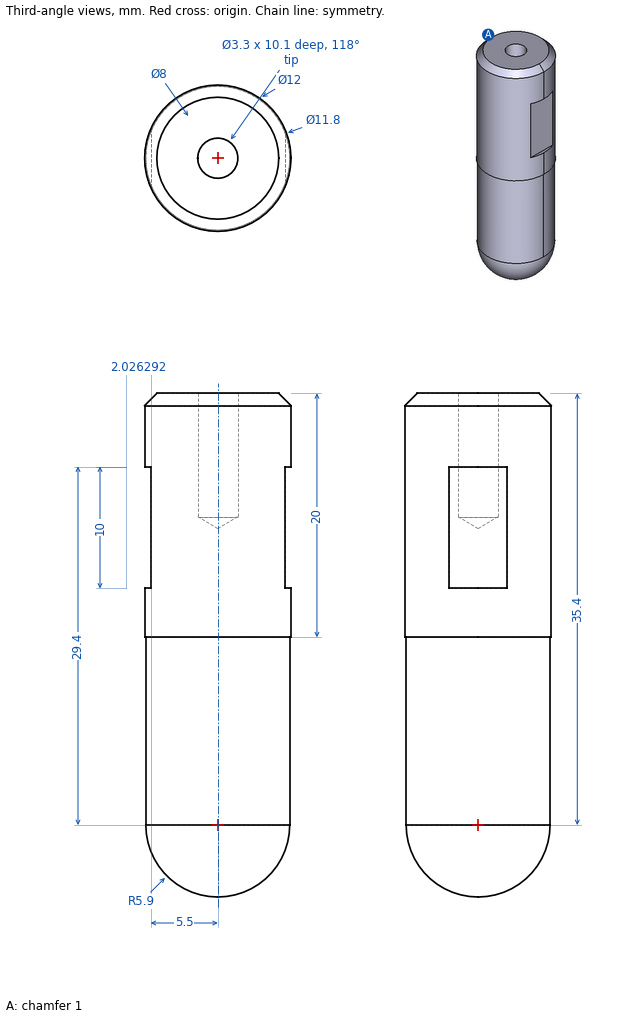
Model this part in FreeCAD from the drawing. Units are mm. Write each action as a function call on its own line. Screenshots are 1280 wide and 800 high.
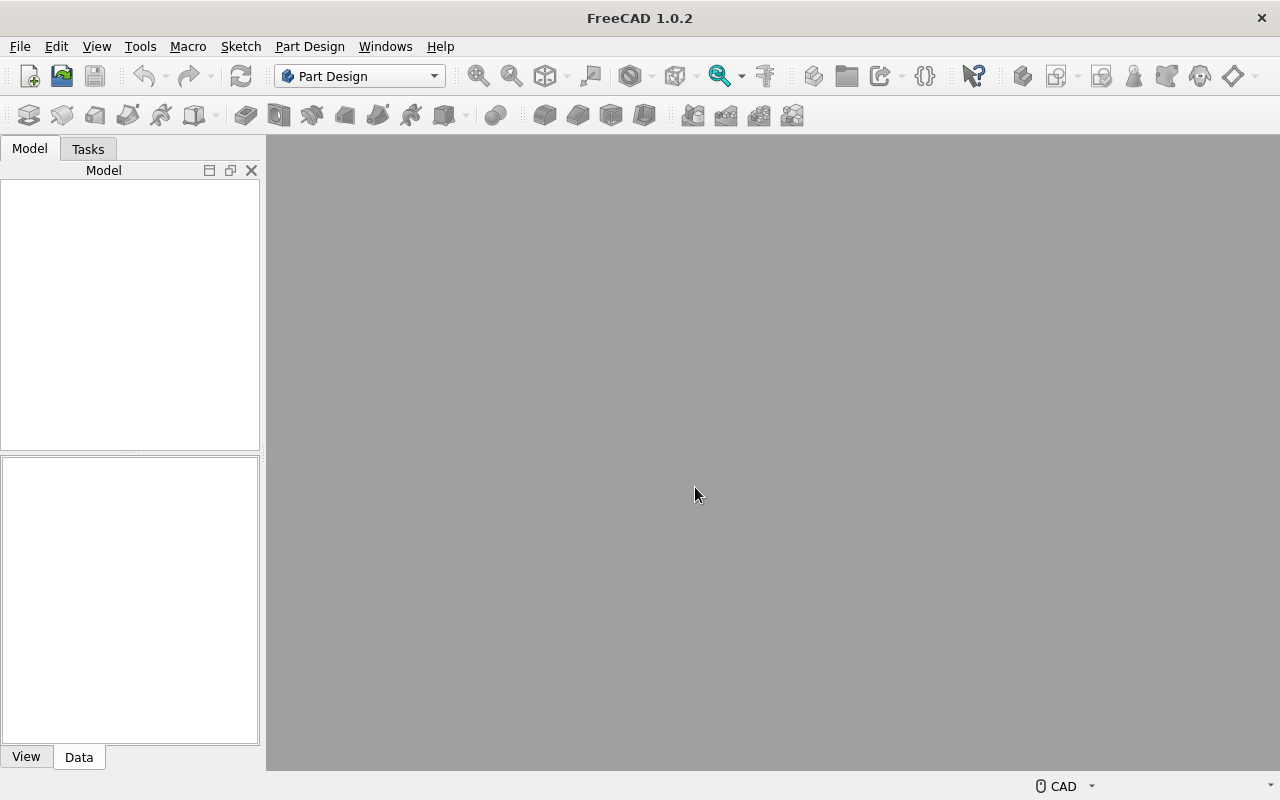
click(29, 76)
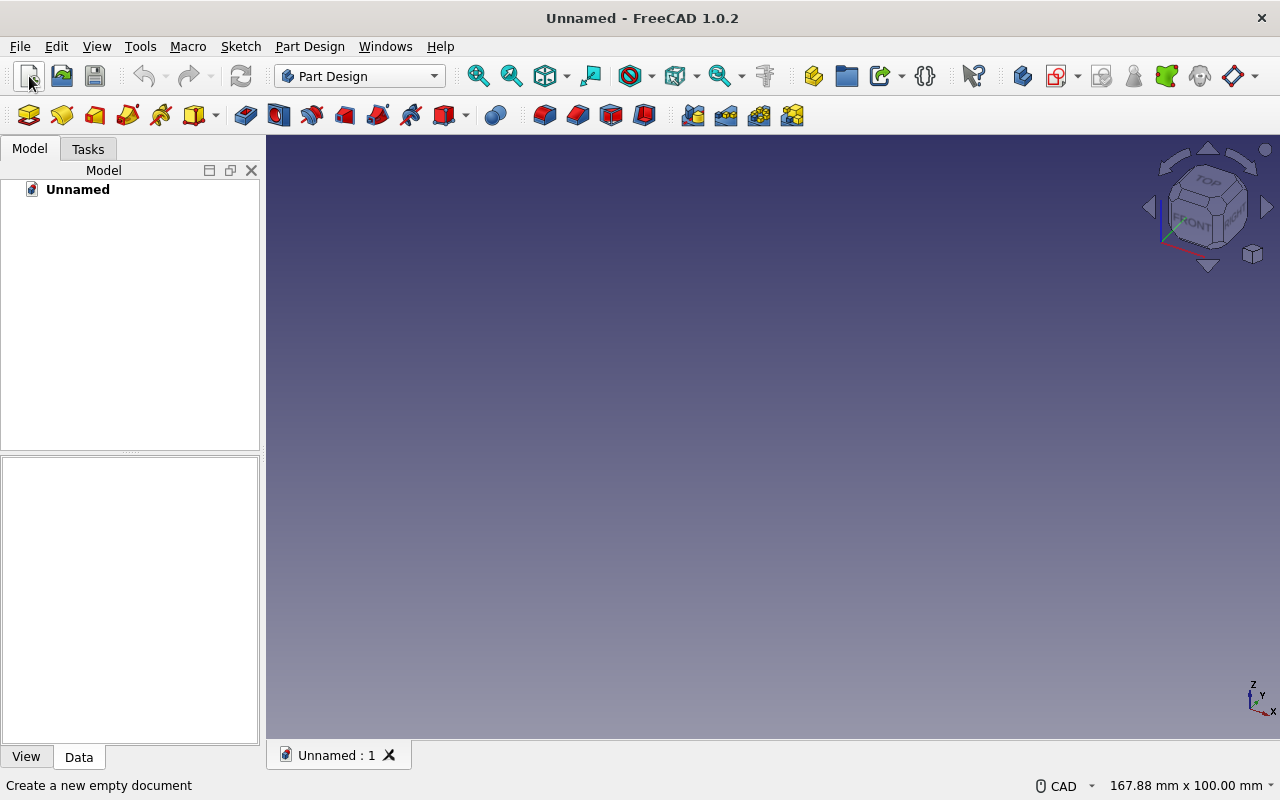
click(1056, 76)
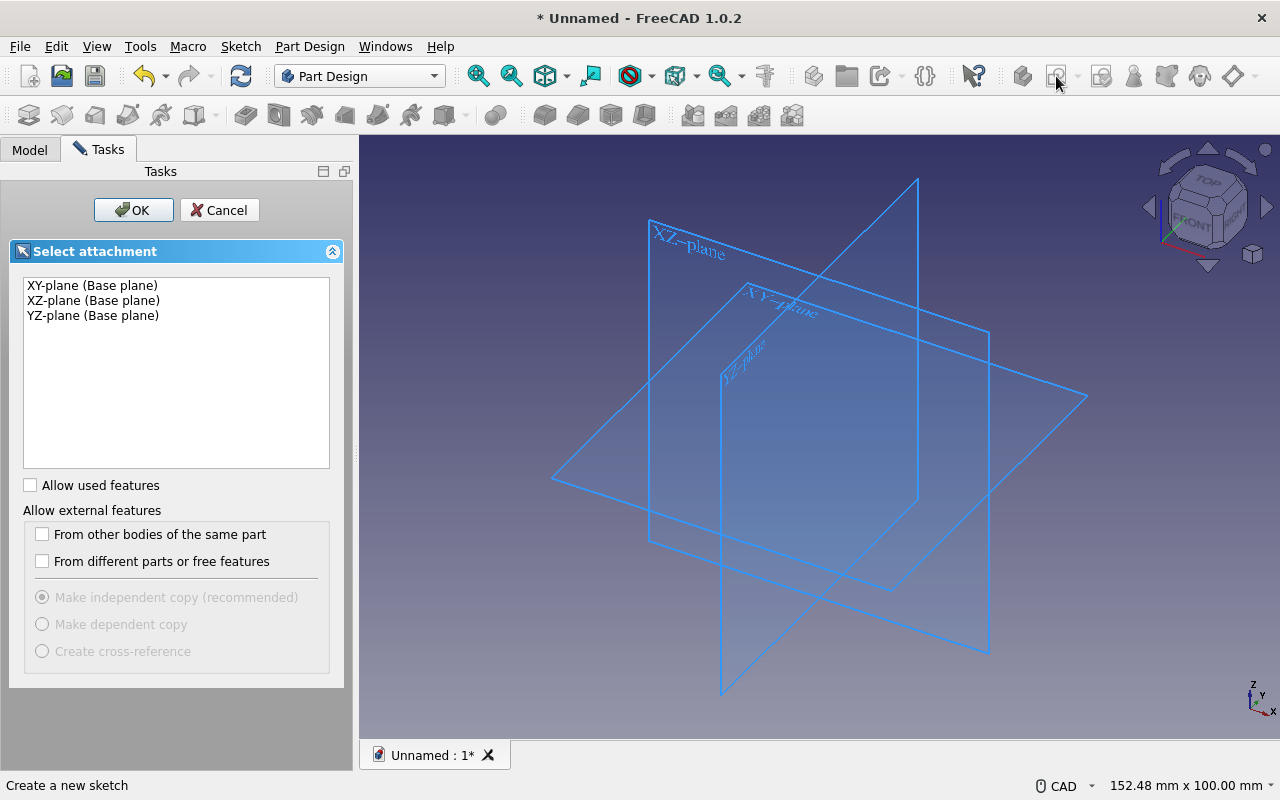
click(84, 286)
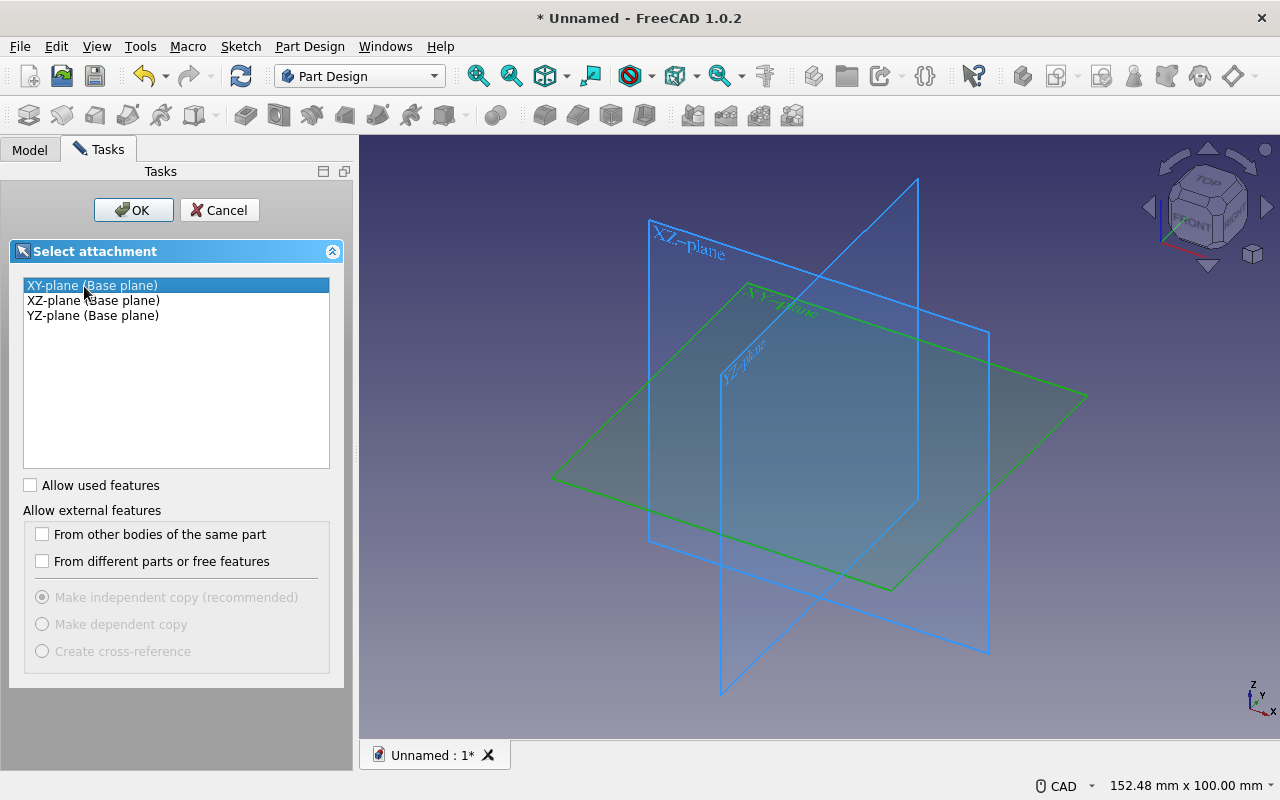
click(134, 210)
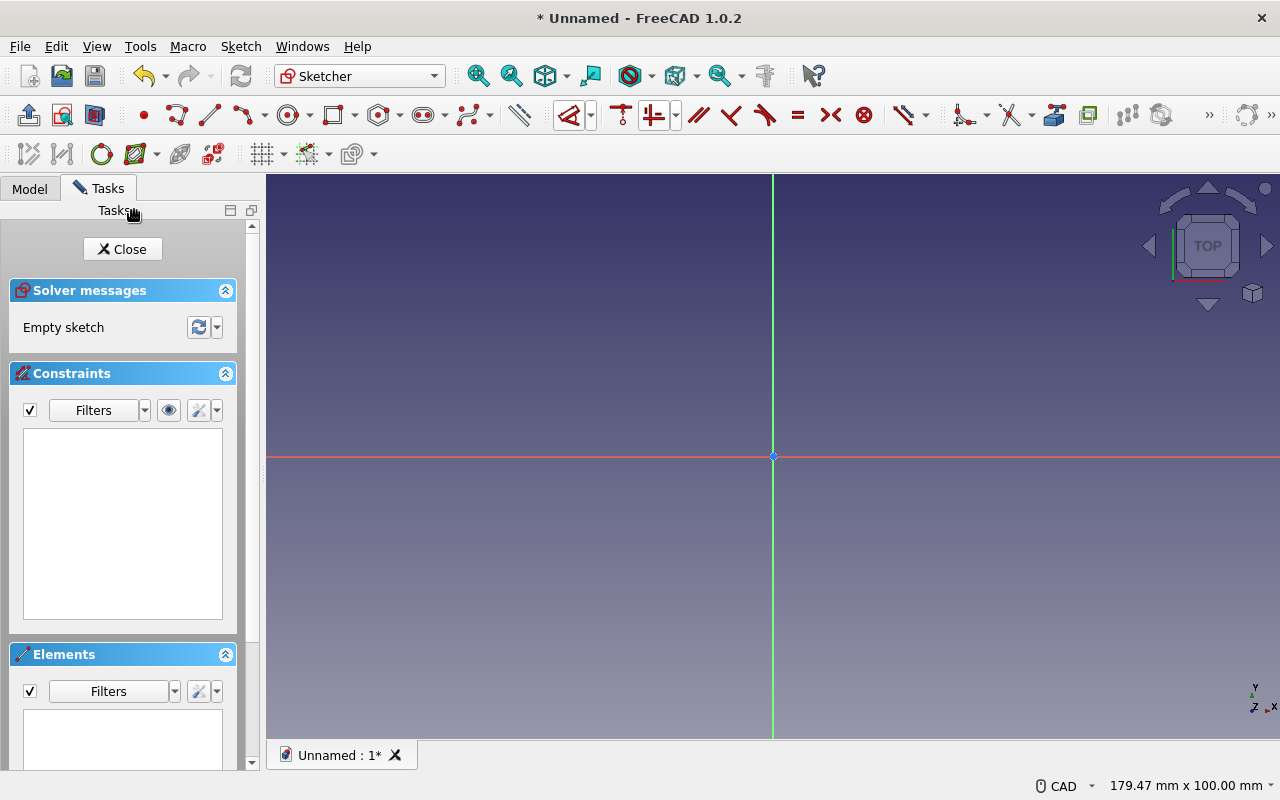
scroll(790, 456, up, 8)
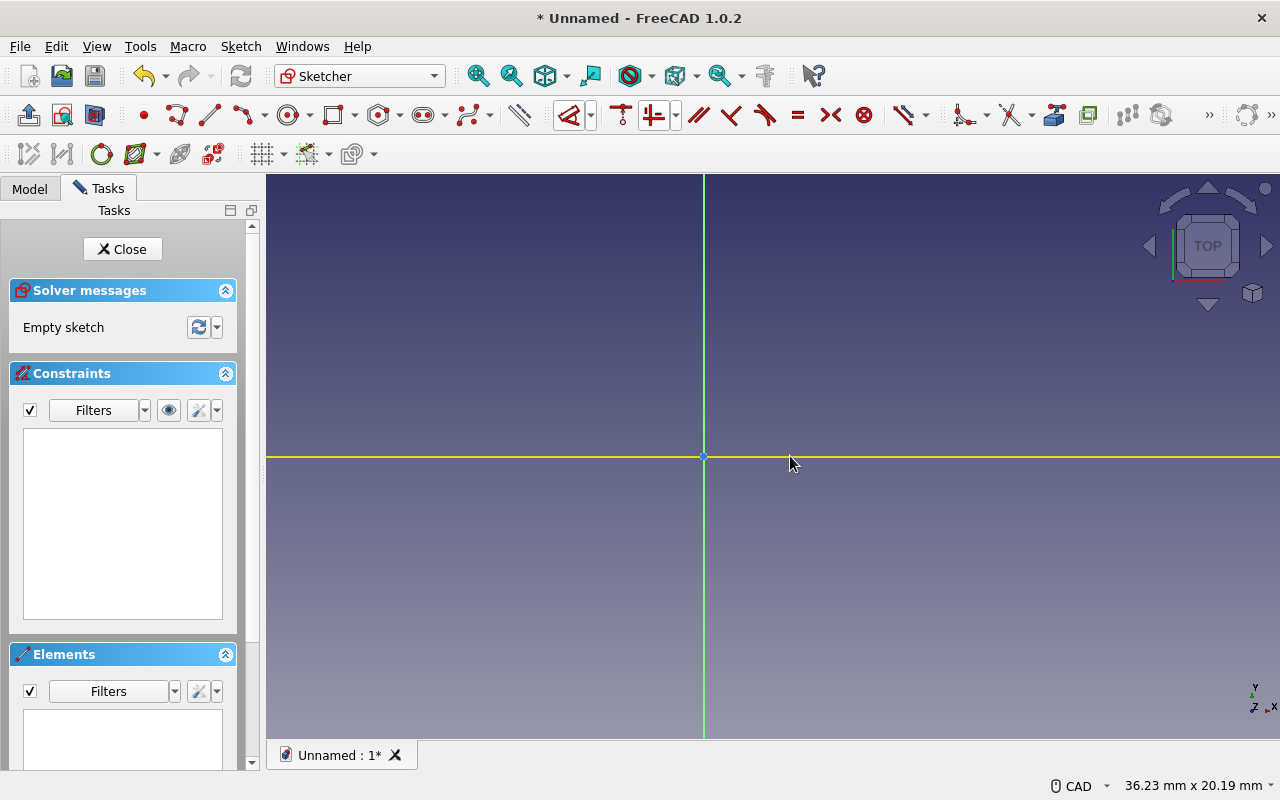
click(288, 116)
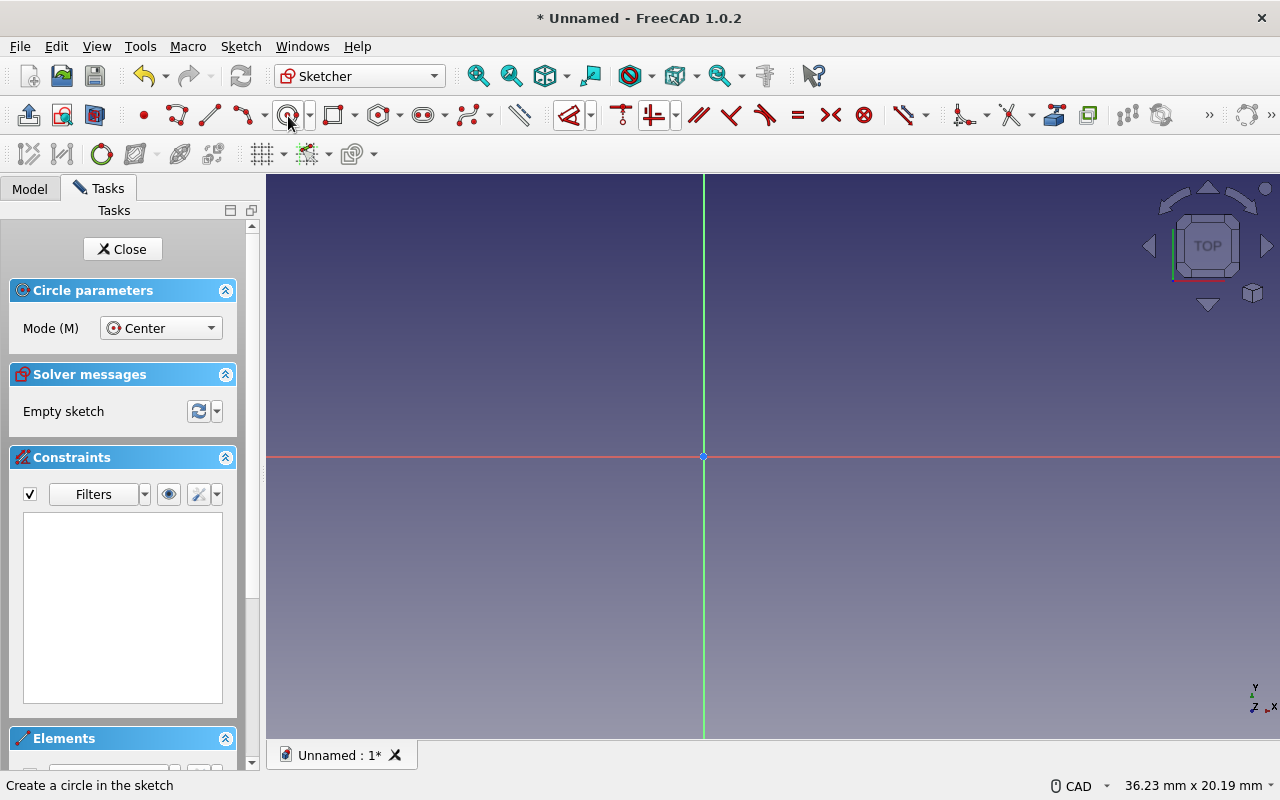
click(704, 456)
click(821, 340)
key(Escape)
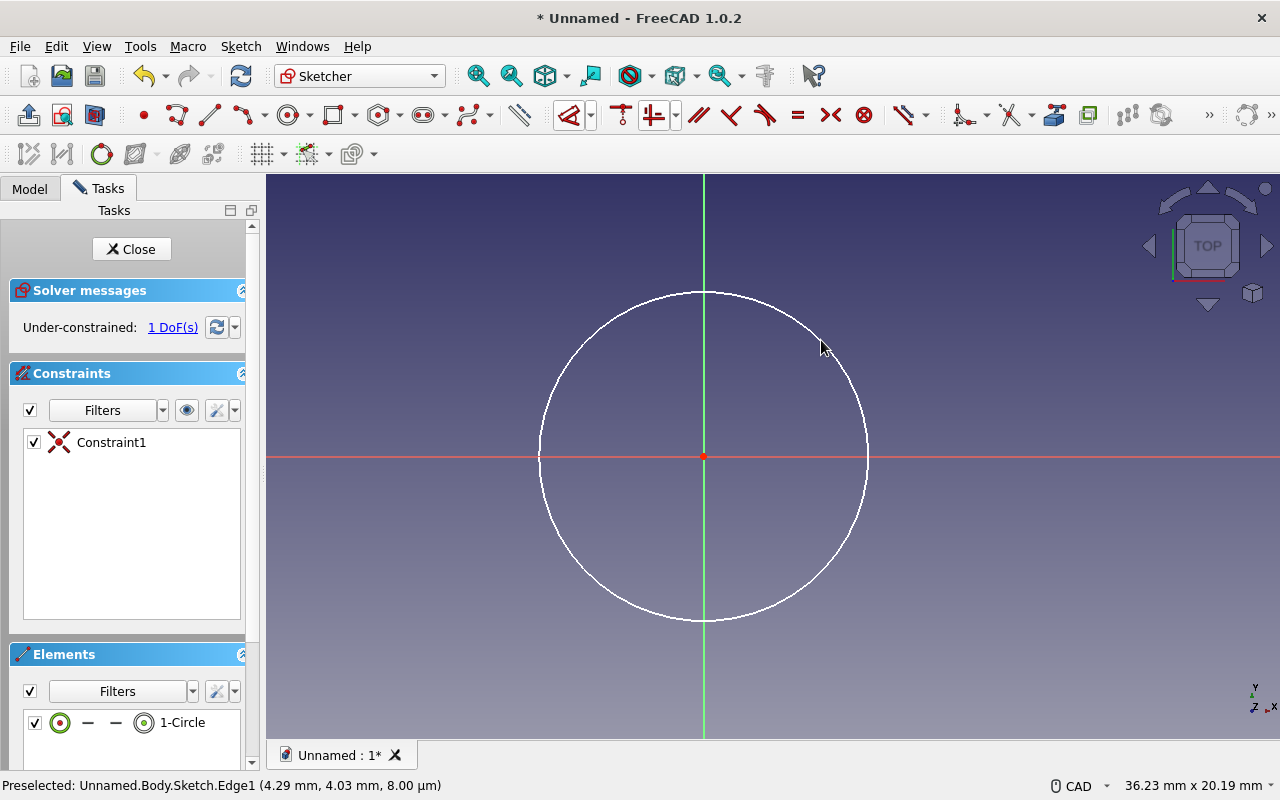
click(568, 116)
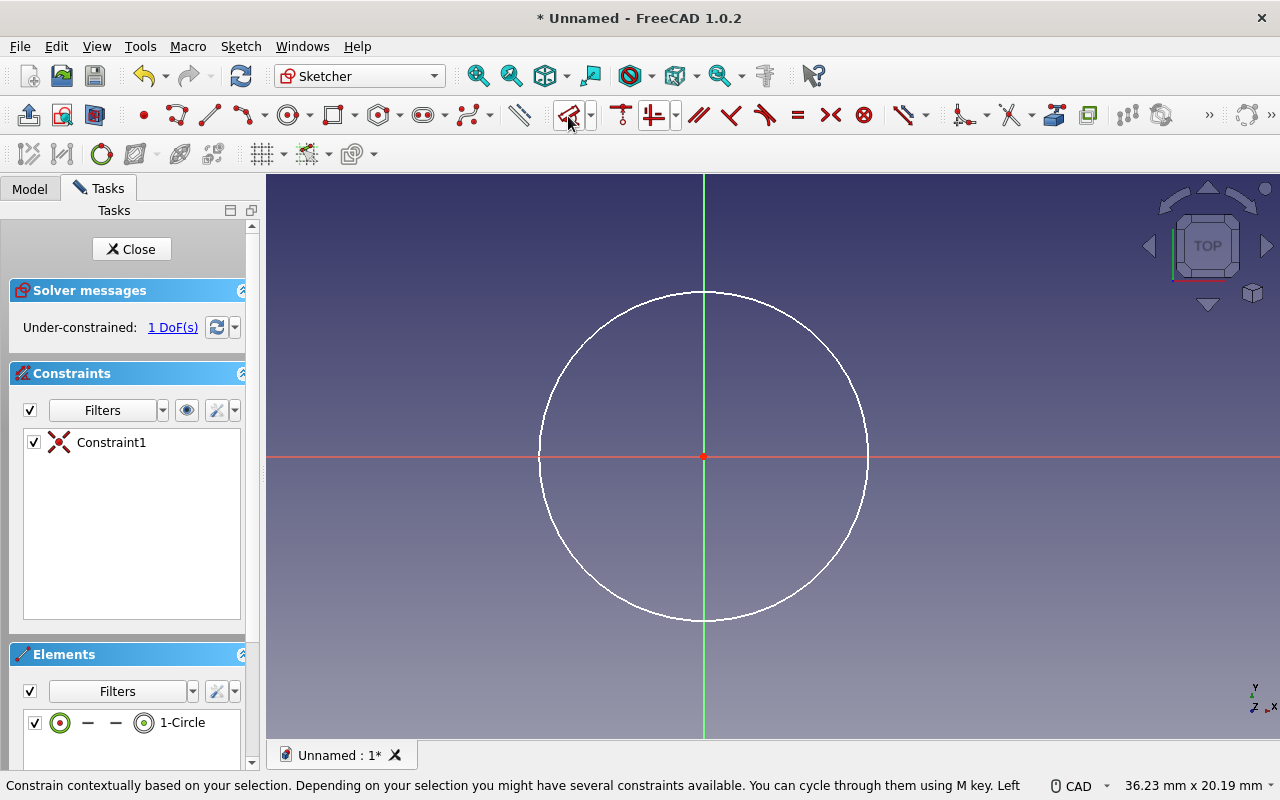
click(820, 340)
click(843, 317)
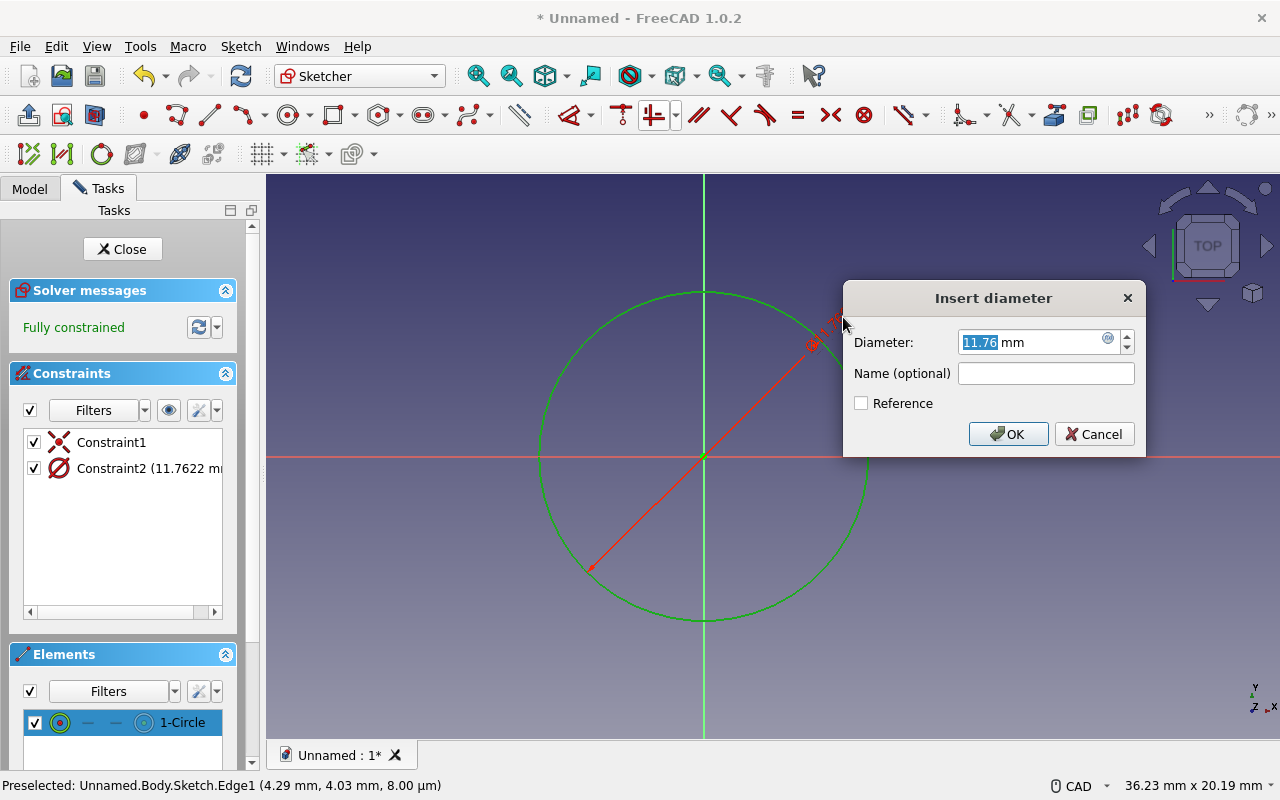
text(11.8)
key(Return)
key(Escape)